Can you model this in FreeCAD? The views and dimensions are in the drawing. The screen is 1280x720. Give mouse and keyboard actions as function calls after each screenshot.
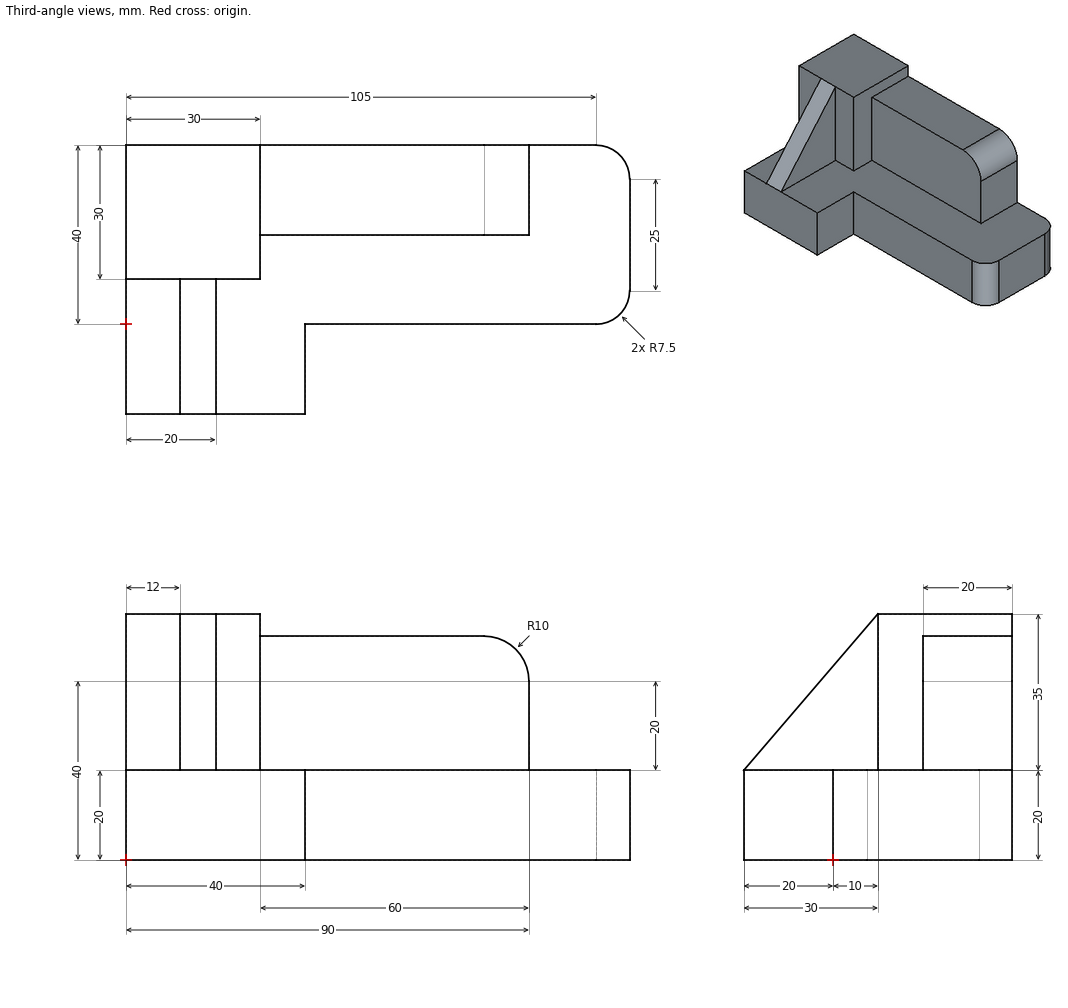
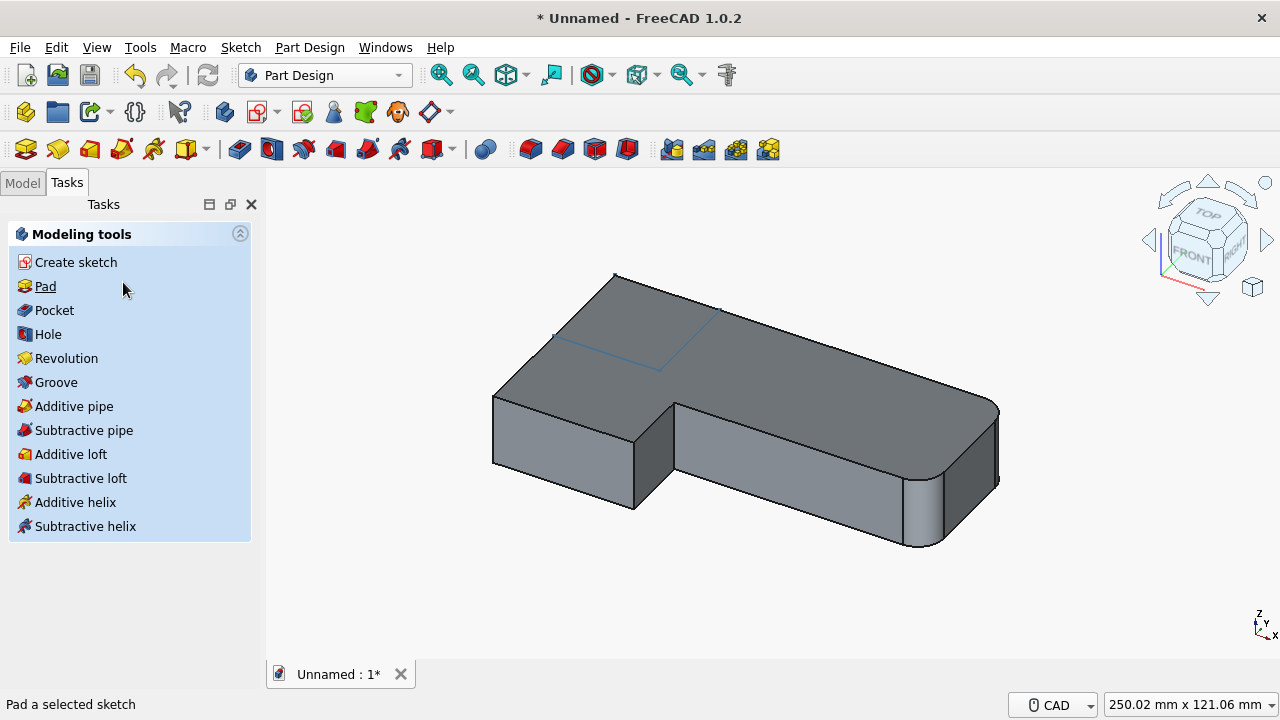
click(26, 150)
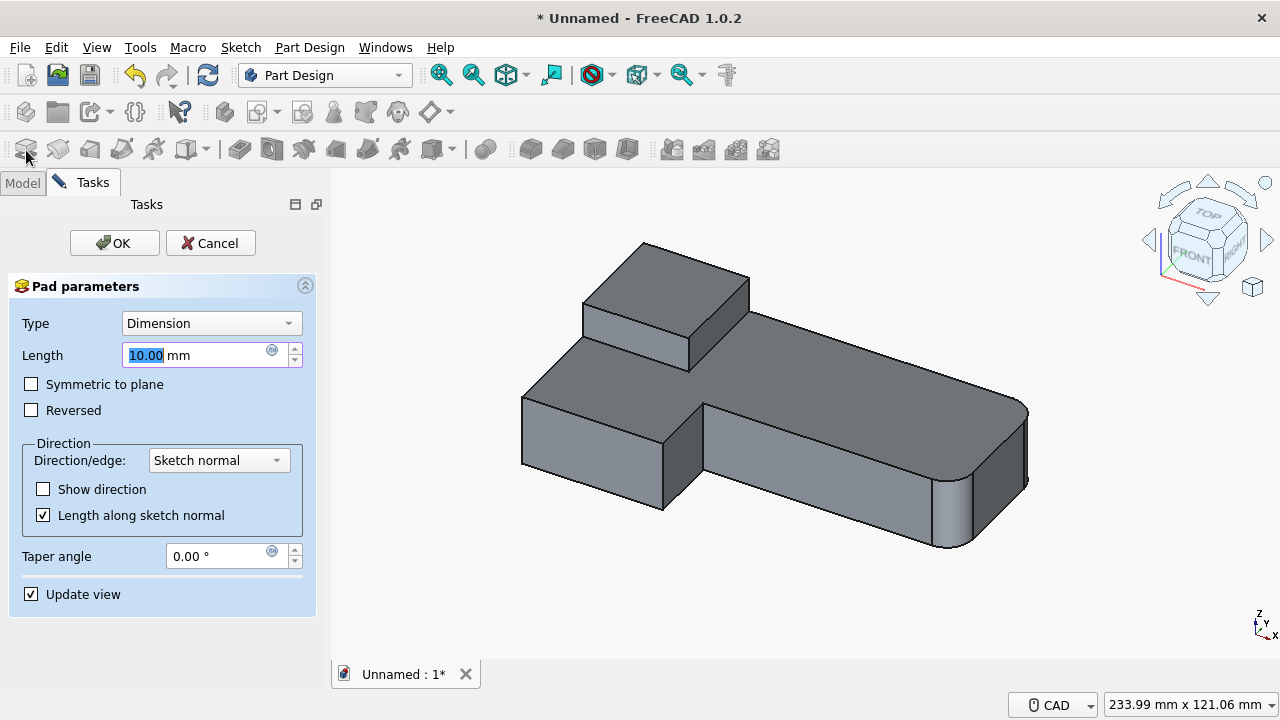
text(35)
key(Tab)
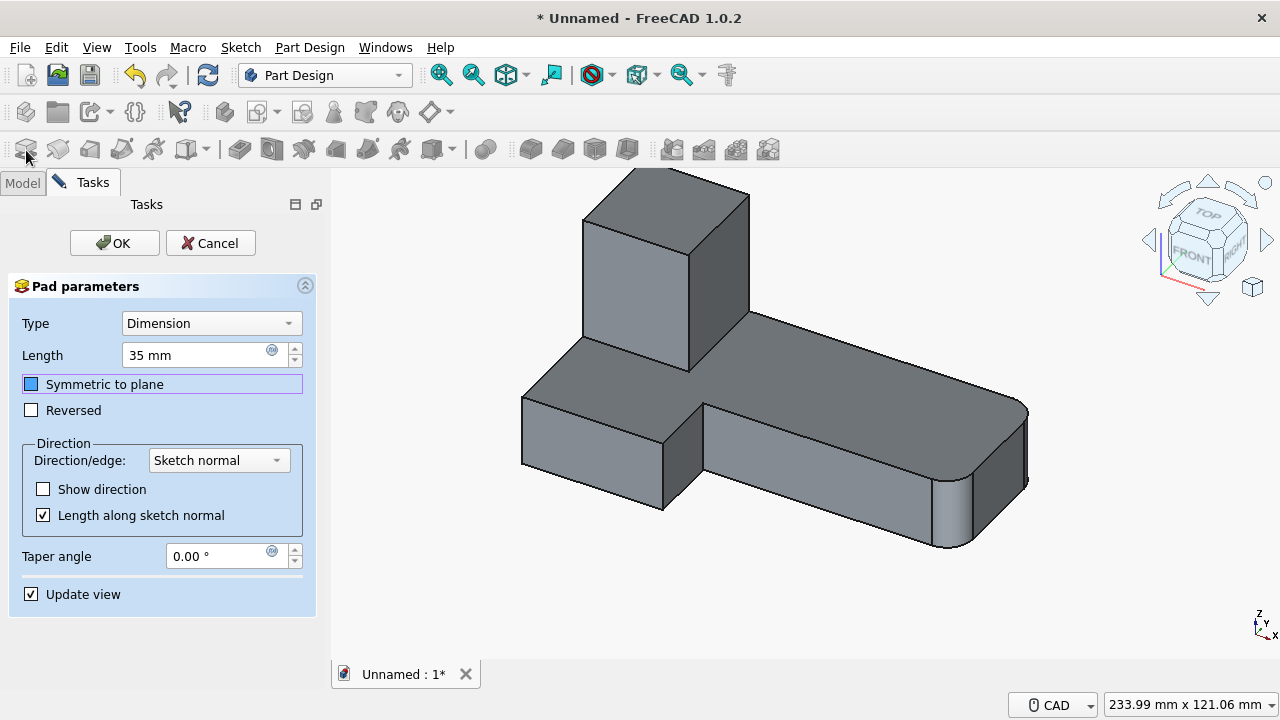
click(115, 243)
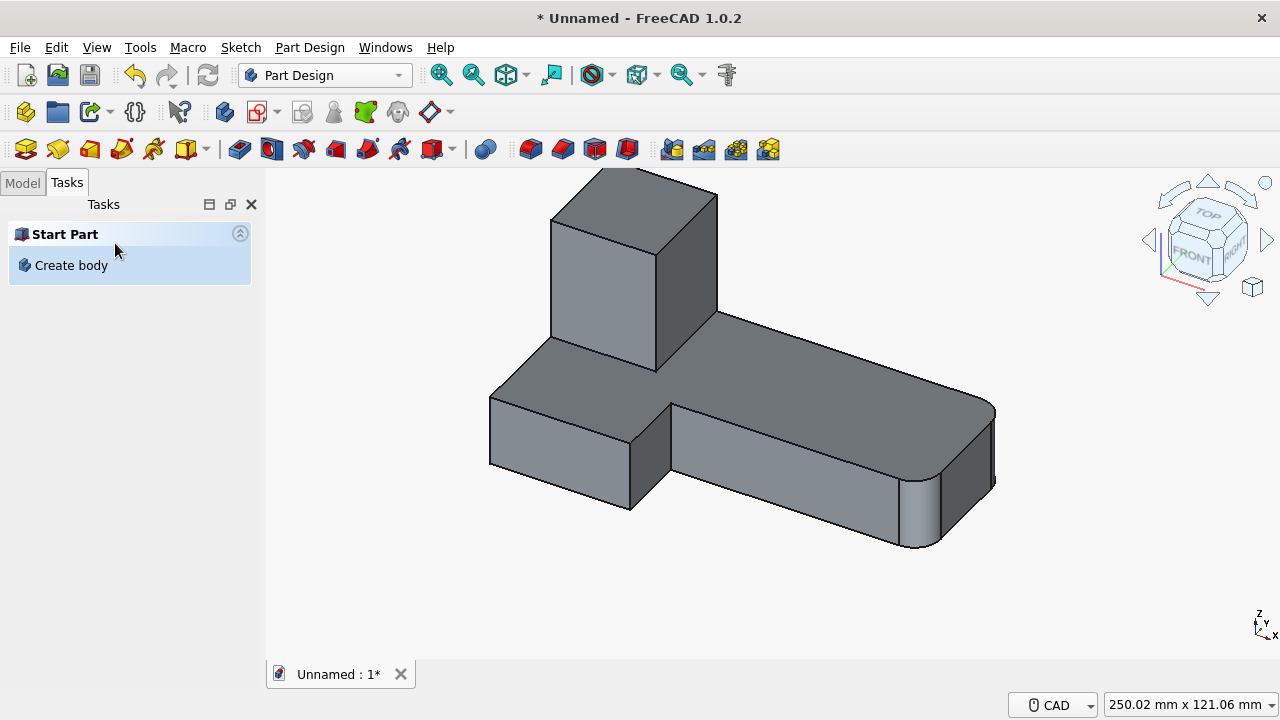
click(442, 76)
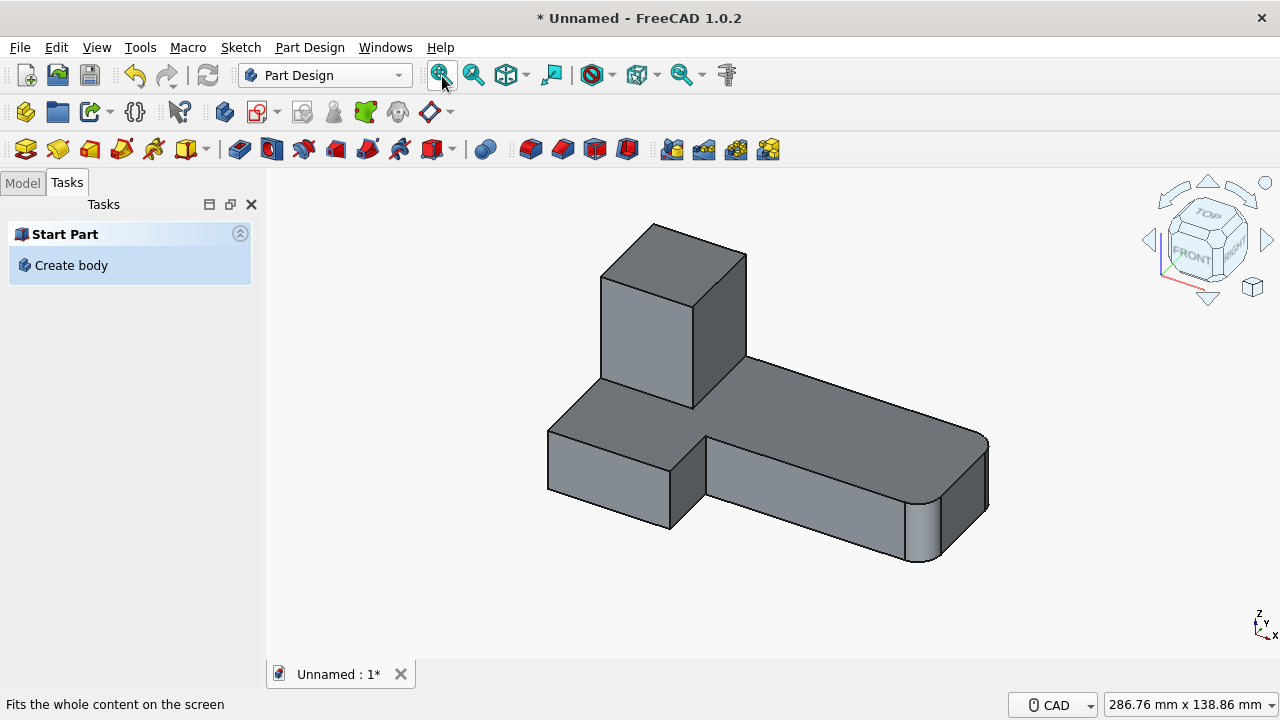
key(4)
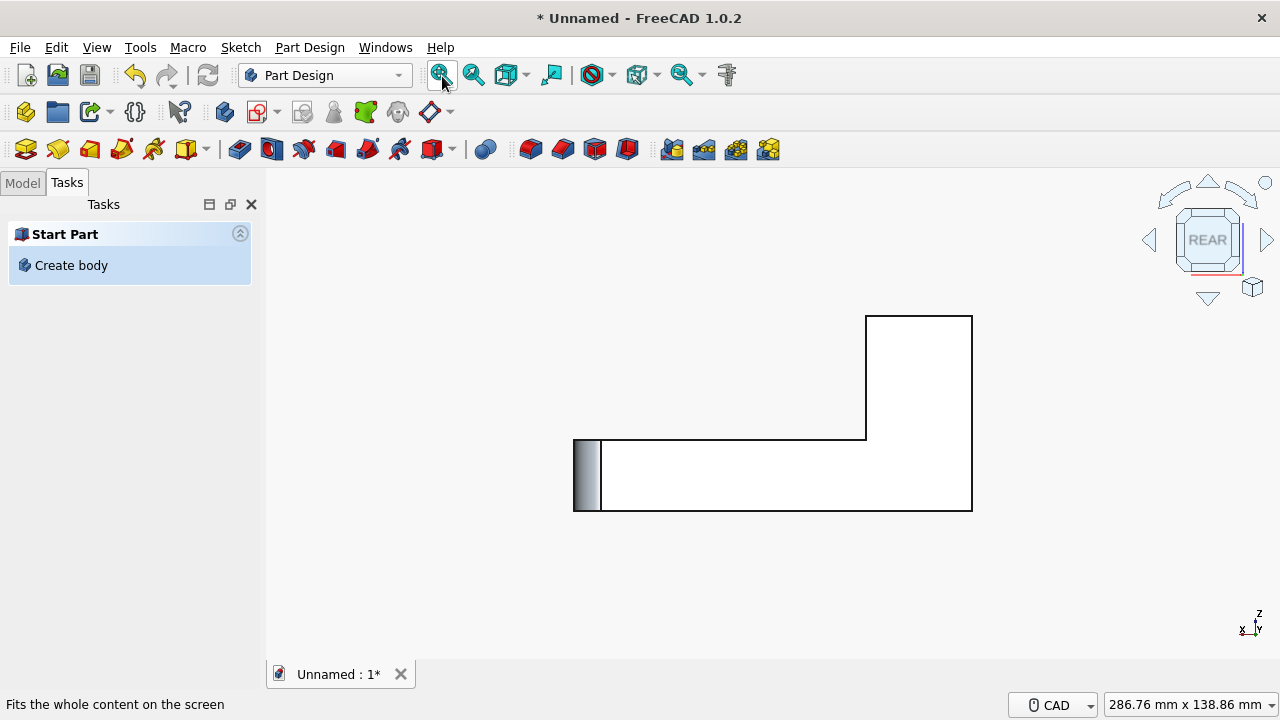
key(v)
key(f)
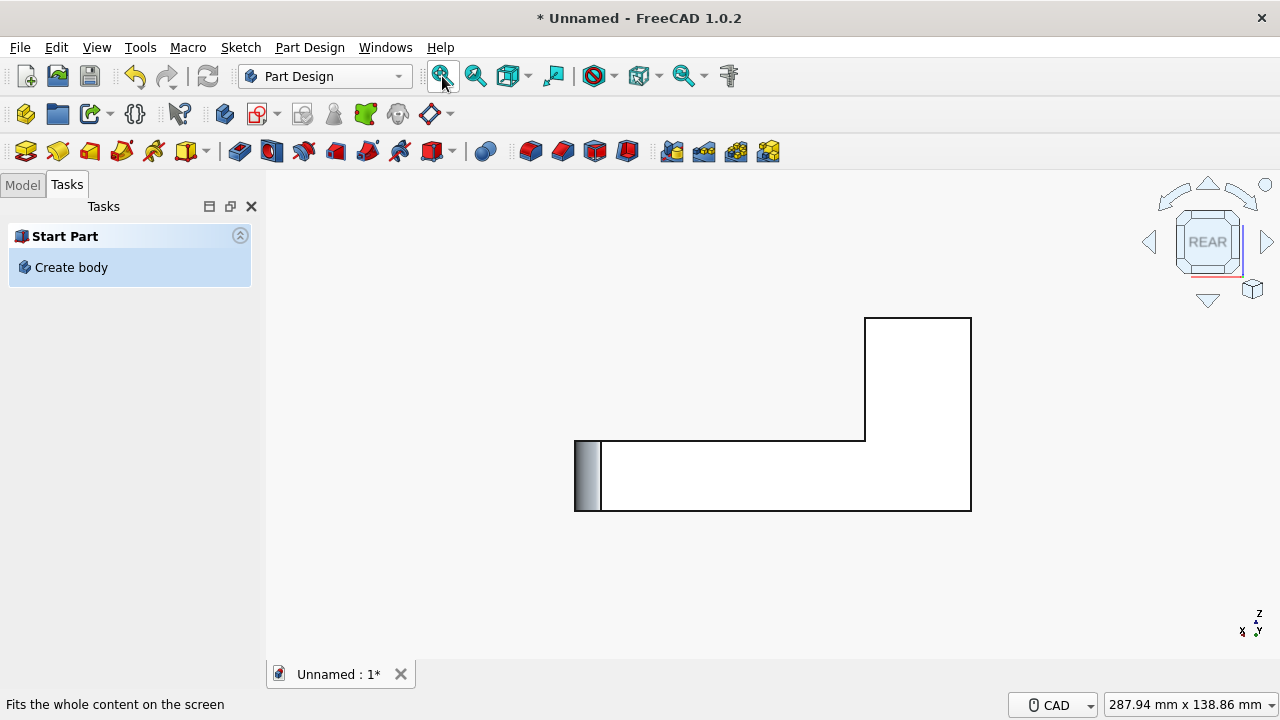
click(892, 469)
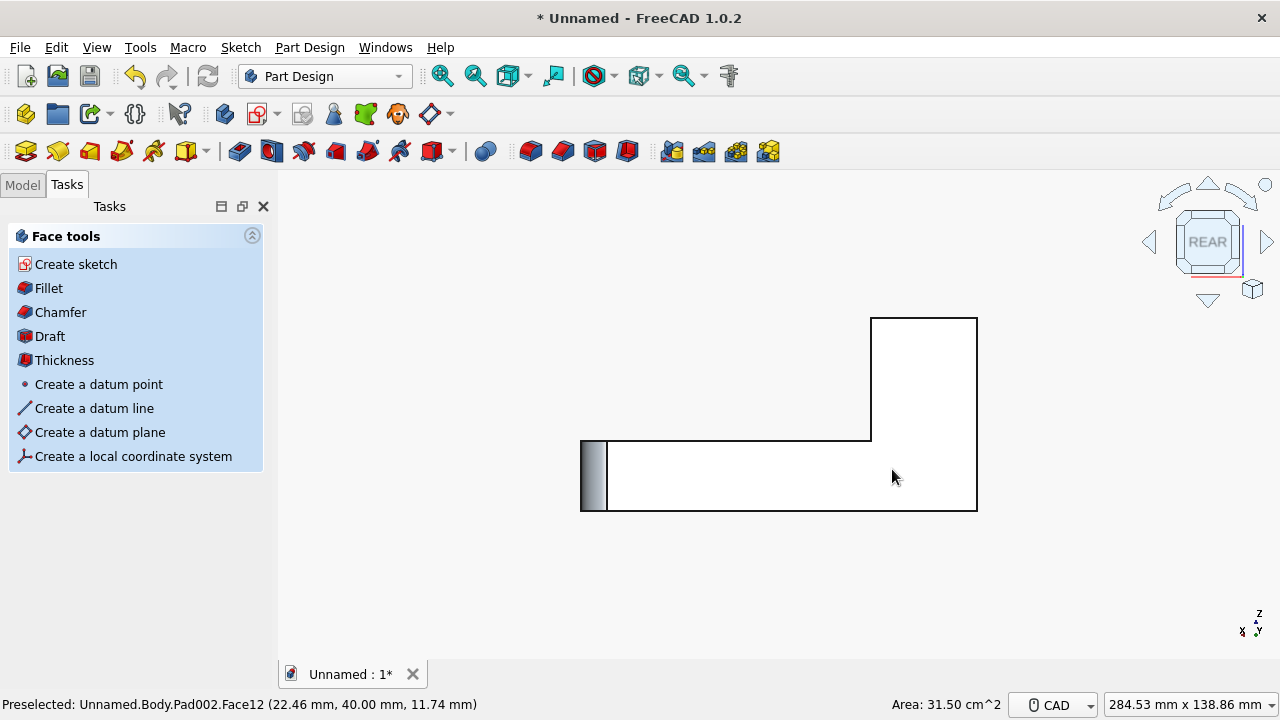
click(258, 114)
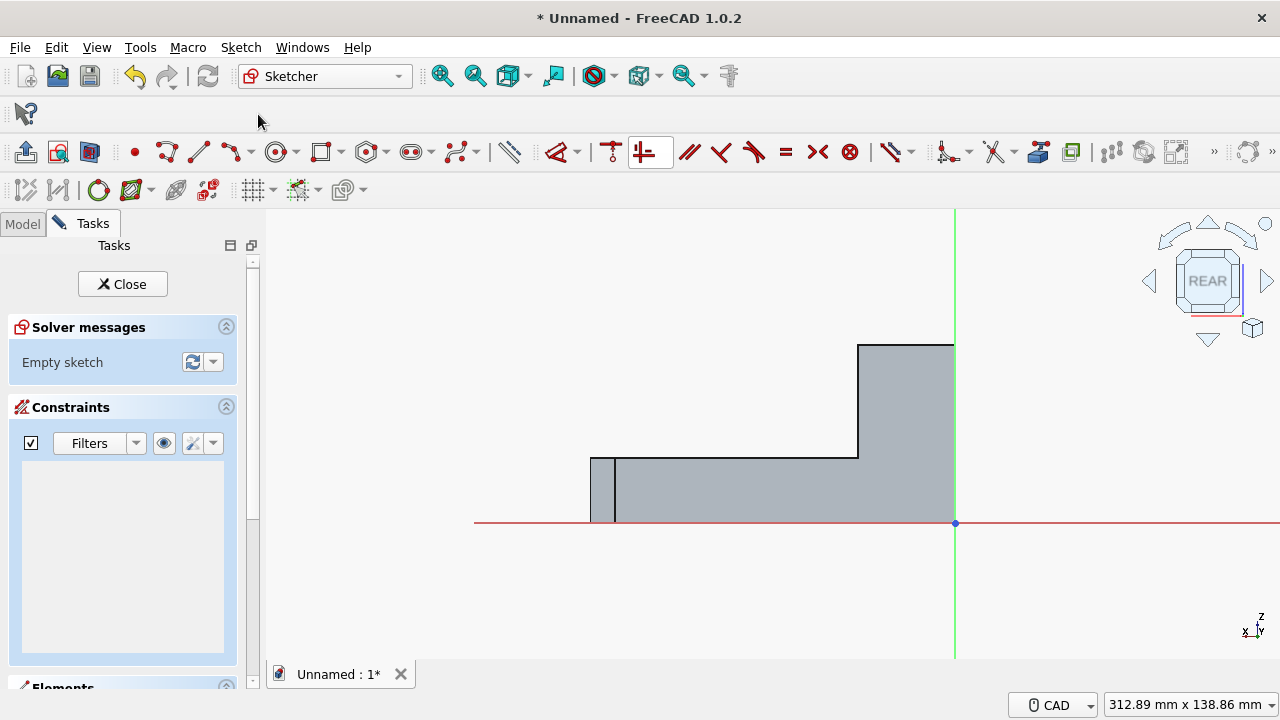
scroll(937, 452, up, 3)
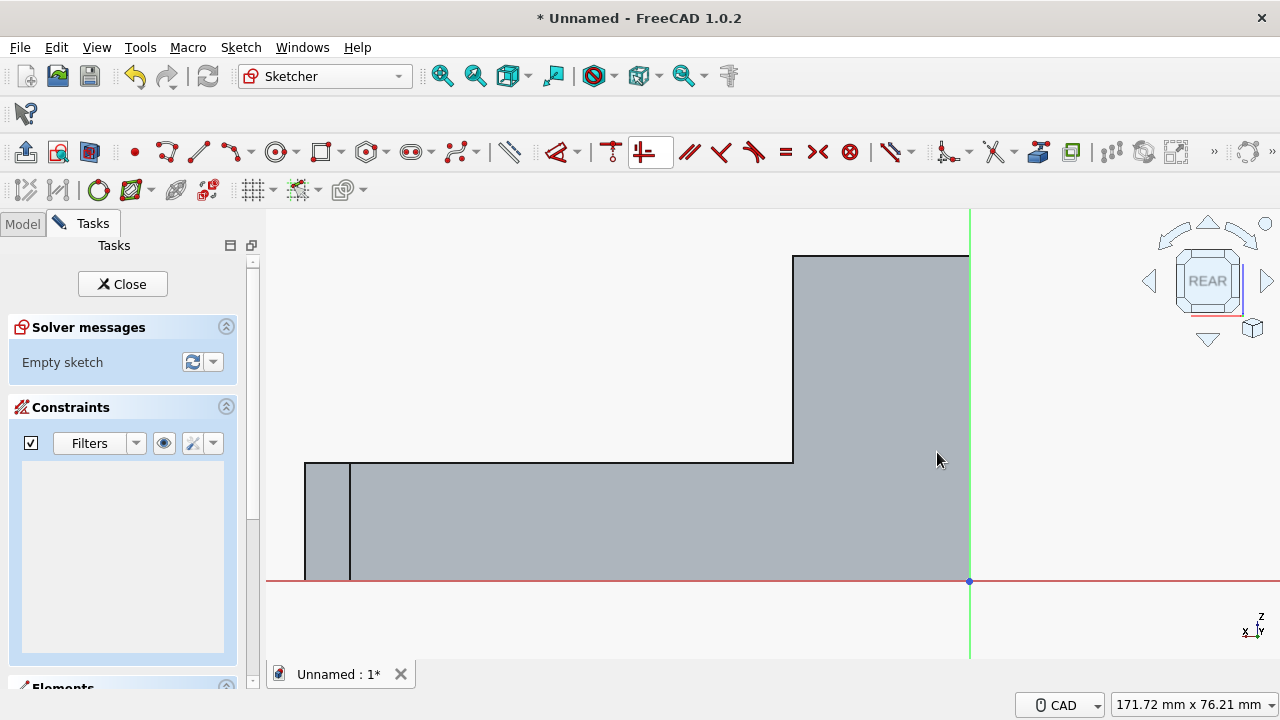
key(g)
key(m)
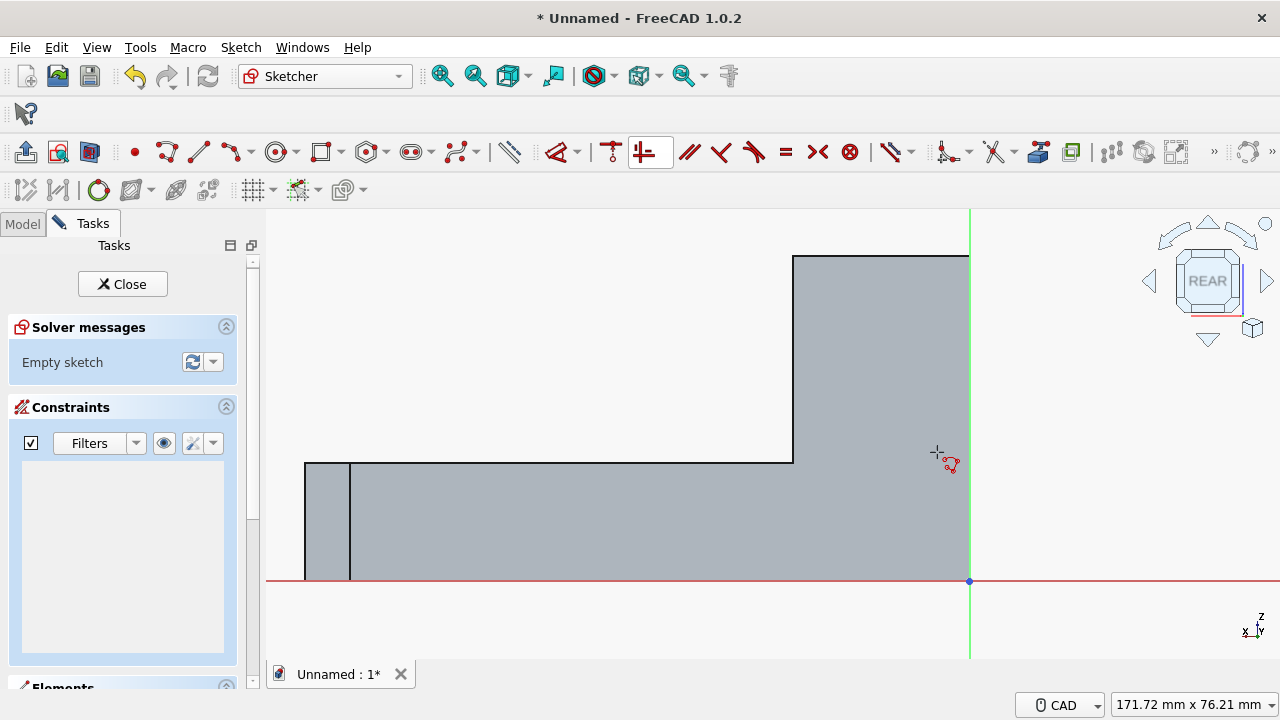
click(438, 345)
click(438, 463)
click(793, 463)
click(793, 286)
click(497, 286)
right_click(497, 286)